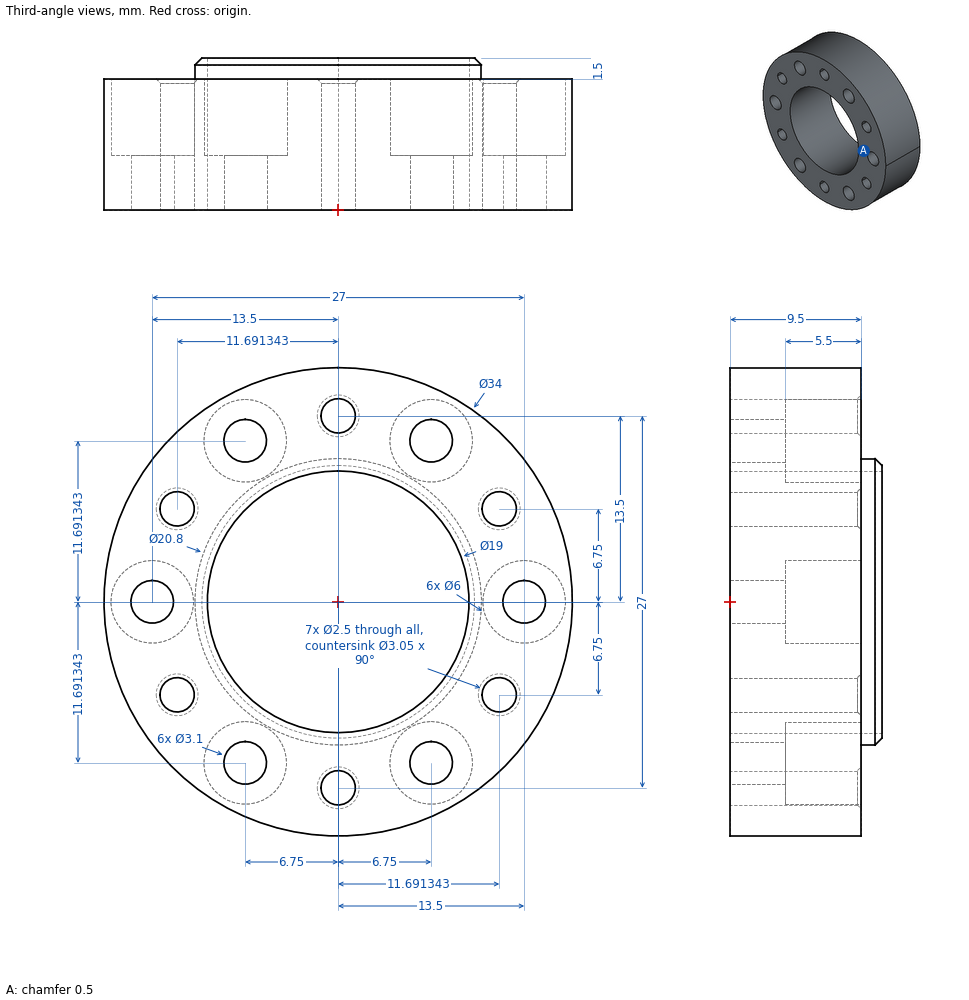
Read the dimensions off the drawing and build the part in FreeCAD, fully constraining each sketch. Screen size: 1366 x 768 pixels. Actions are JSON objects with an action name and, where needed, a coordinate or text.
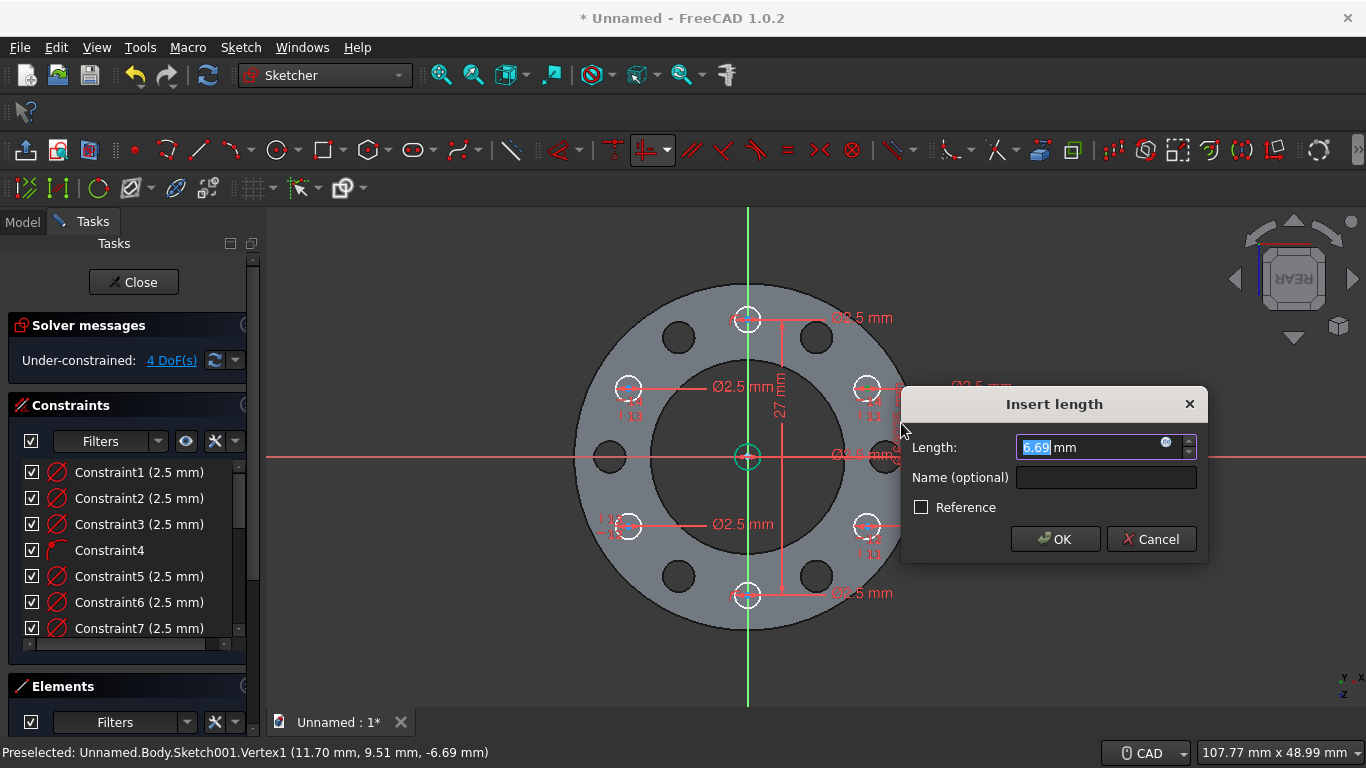
{"action": "type", "text": "6.75"}
{"action": "key", "text": "Return"}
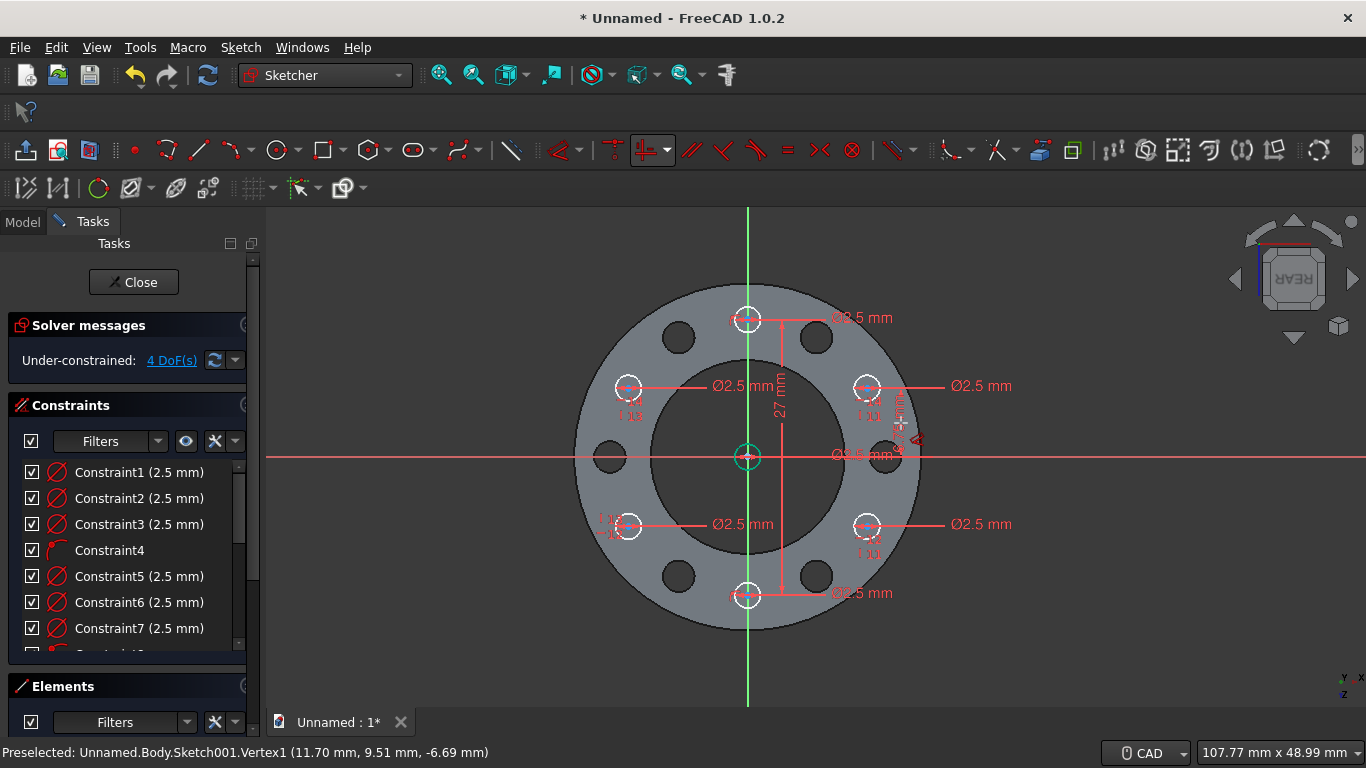
{"action": "left_click", "coordinate": [867, 526]}
{"action": "left_click", "coordinate": [901, 492]}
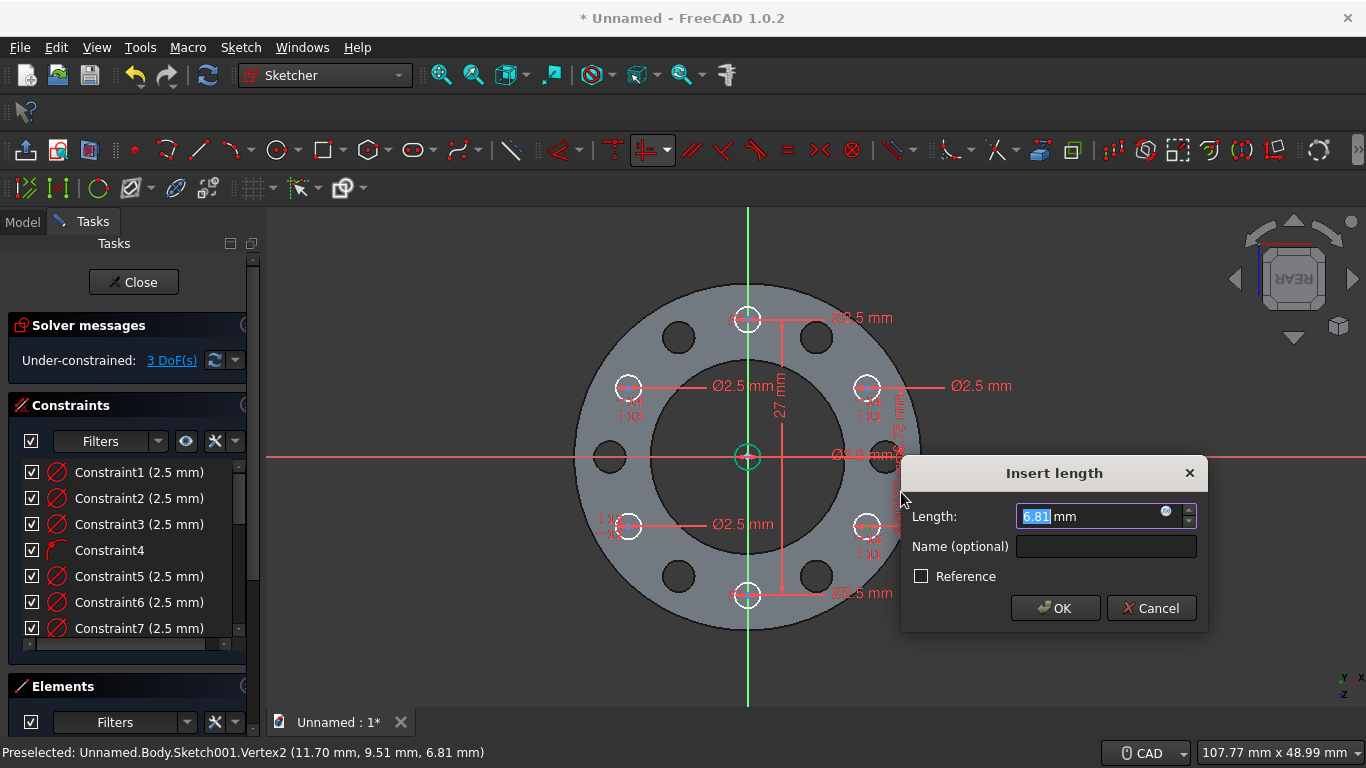
{"action": "type", "text": "6.75"}
{"action": "key", "text": "Return"}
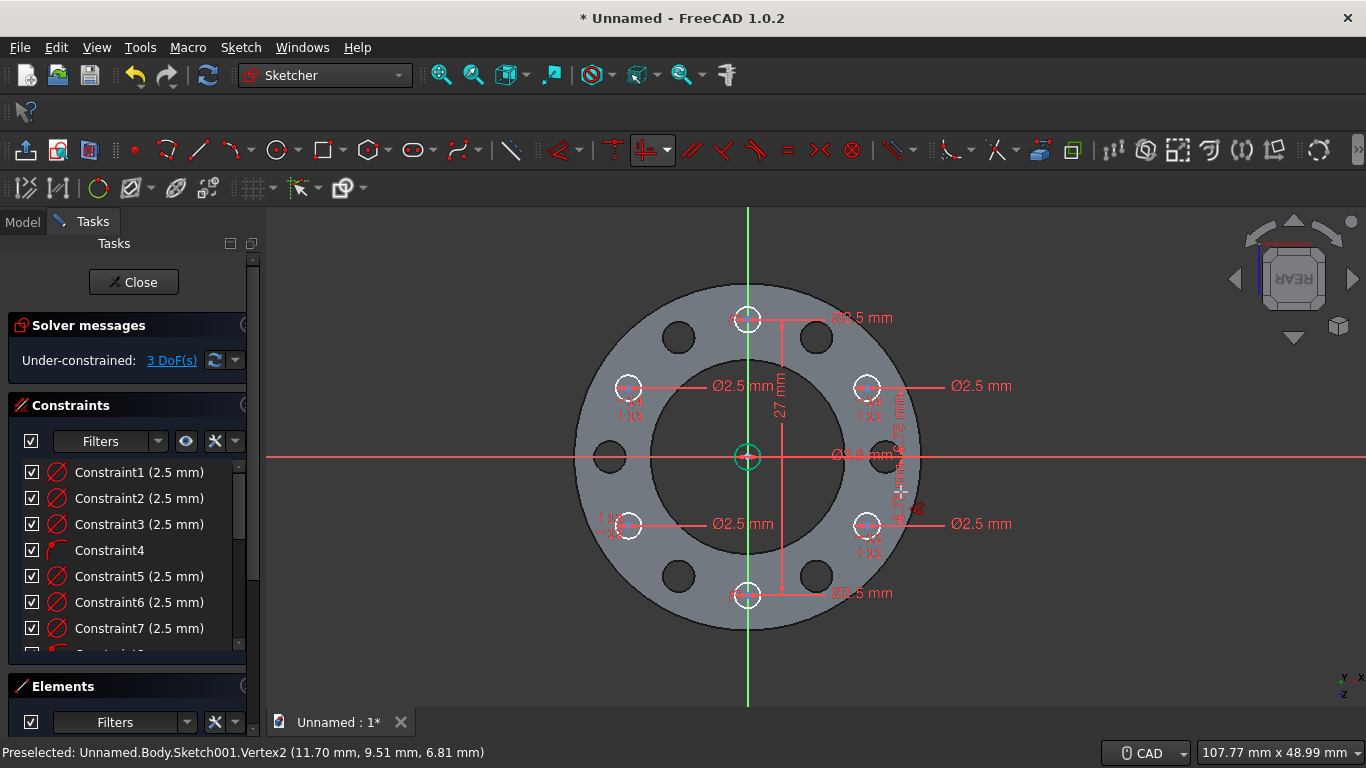
{"action": "left_click", "coordinate": [748, 595]}
{"action": "left_click", "coordinate": [782, 526]}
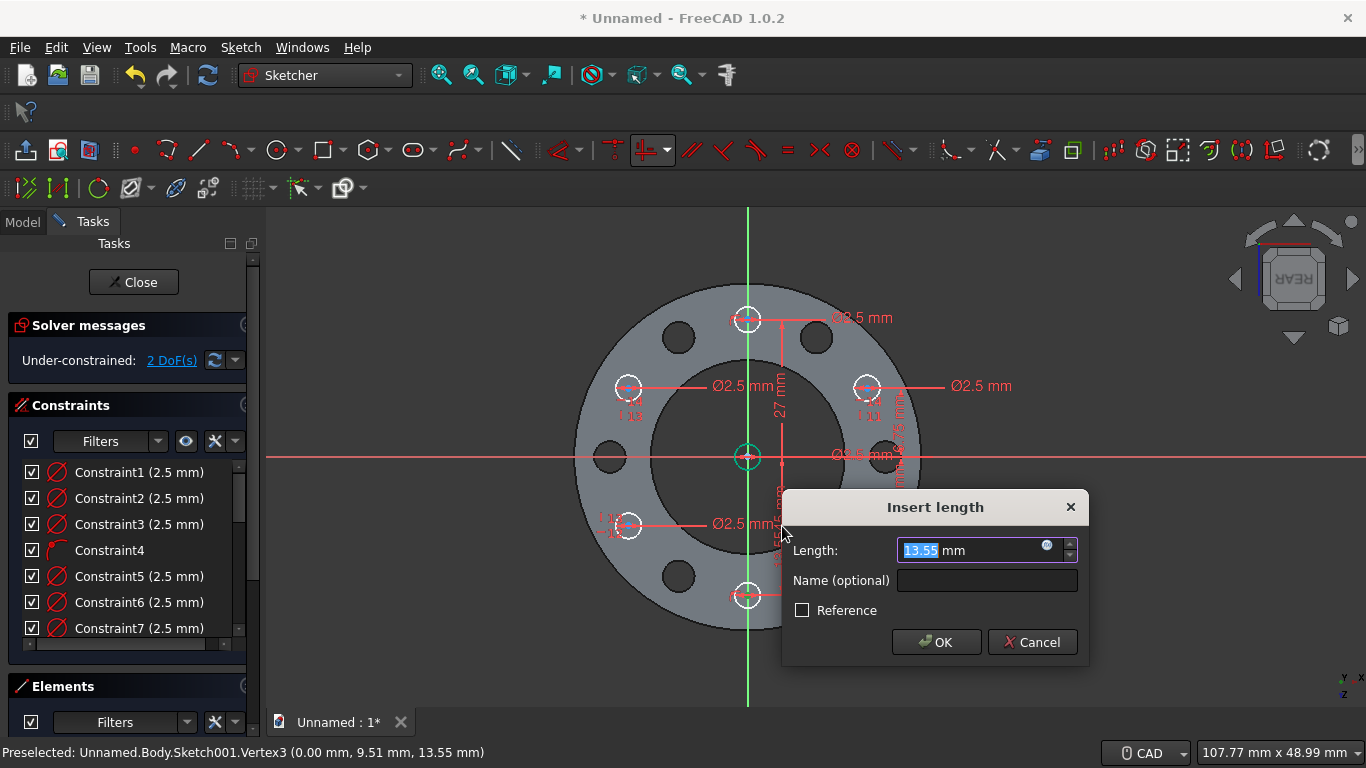
{"action": "type", "text": "13.5"}
{"action": "key", "text": "Return"}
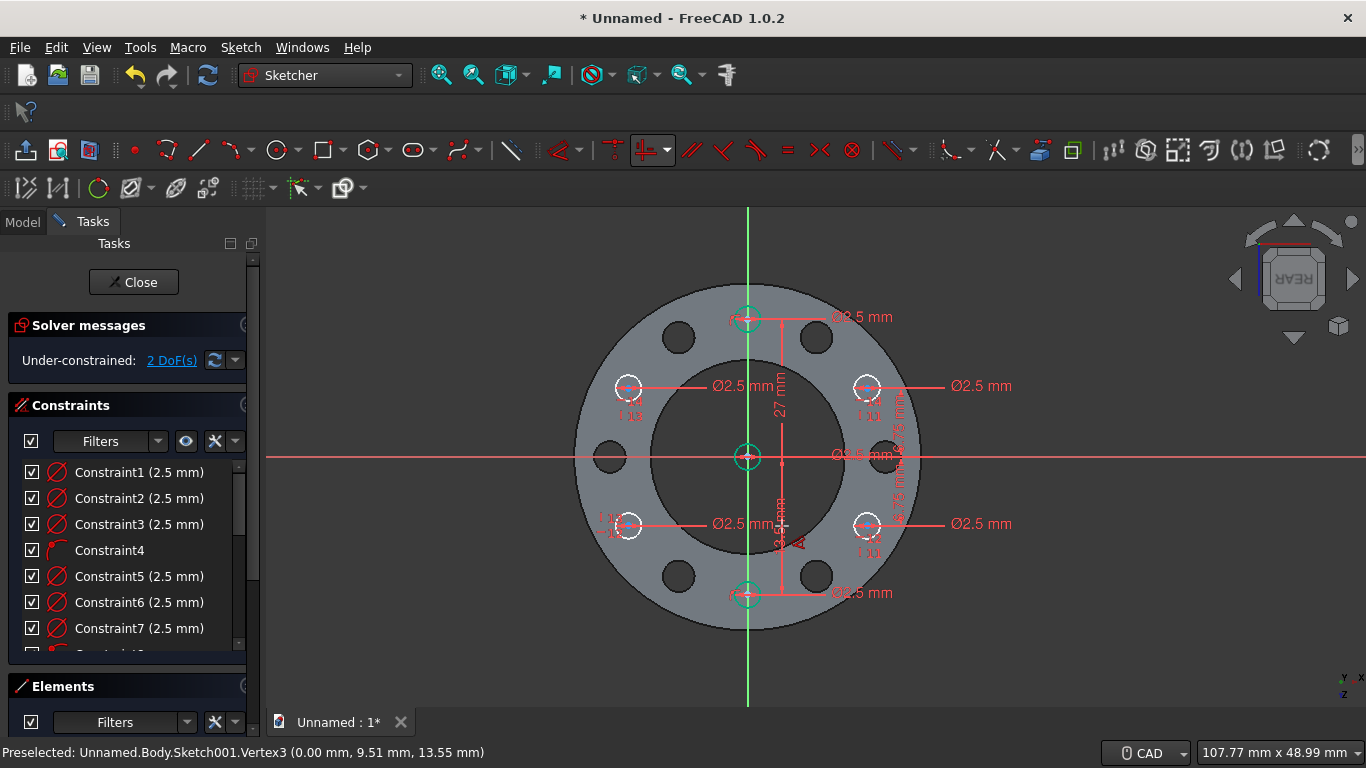
{"action": "left_click", "coordinate": [867, 388]}
{"action": "left_click", "coordinate": [807, 354]}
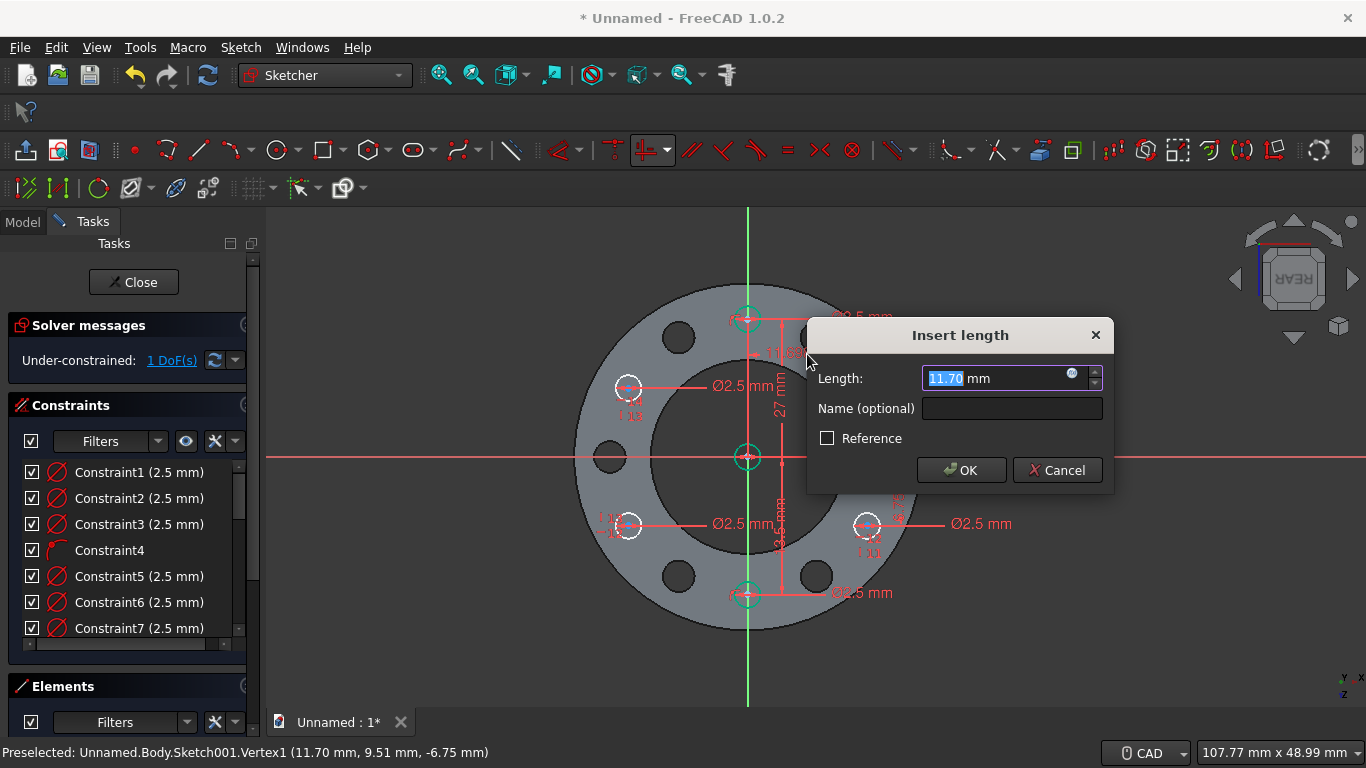
{"action": "type", "text": "11.691343"}
{"action": "key", "text": "Return"}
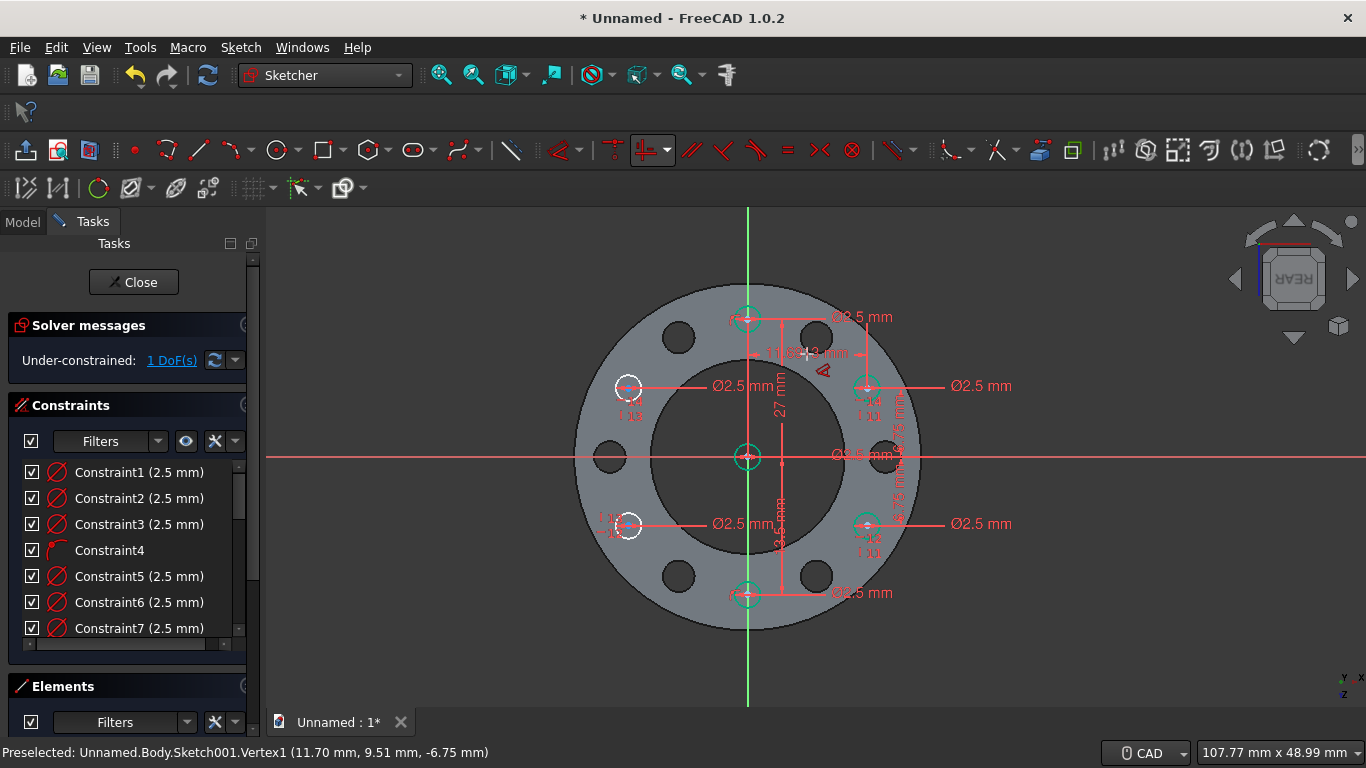
{"action": "left_click", "coordinate": [629, 526]}
{"action": "left_click", "coordinate": [688, 560]}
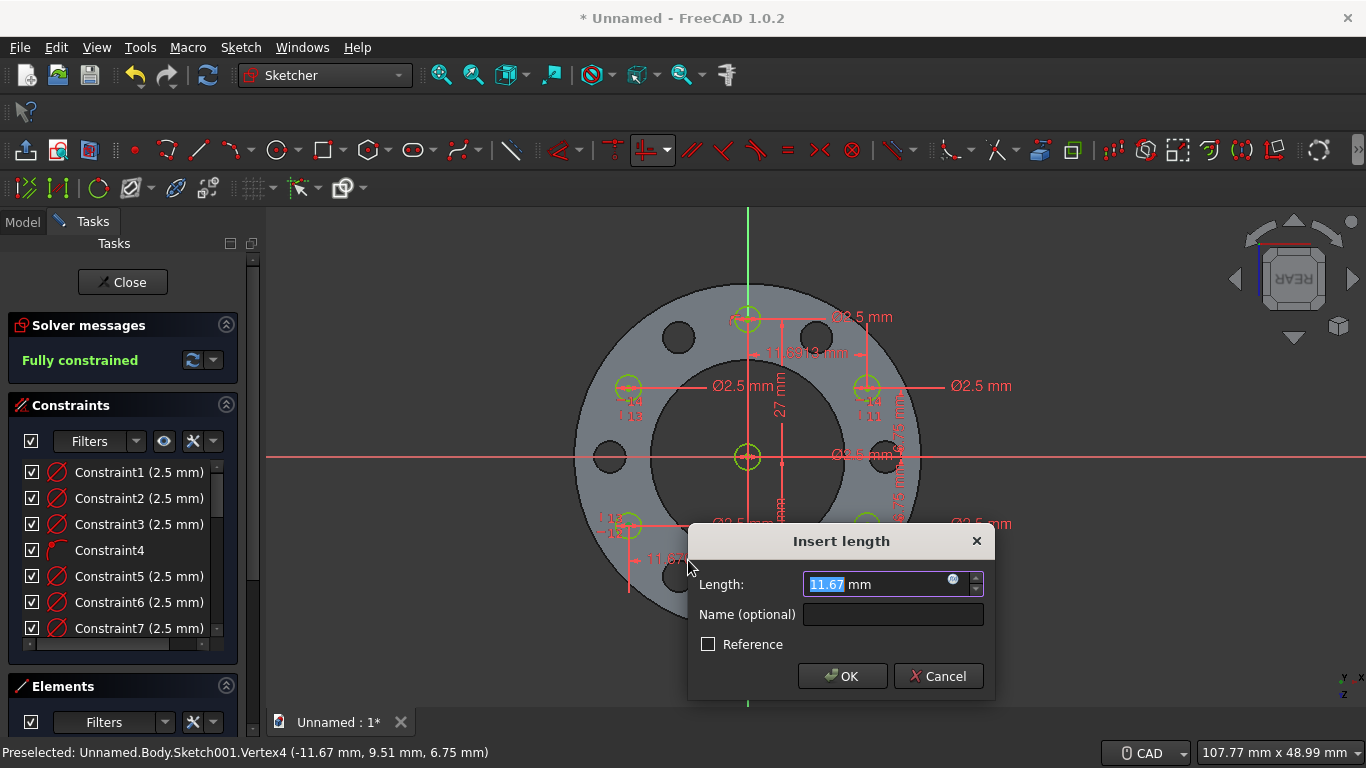
{"action": "type", "text": "11.691343"}
{"action": "key", "text": "Return"}
{"action": "key", "text": "Escape"}